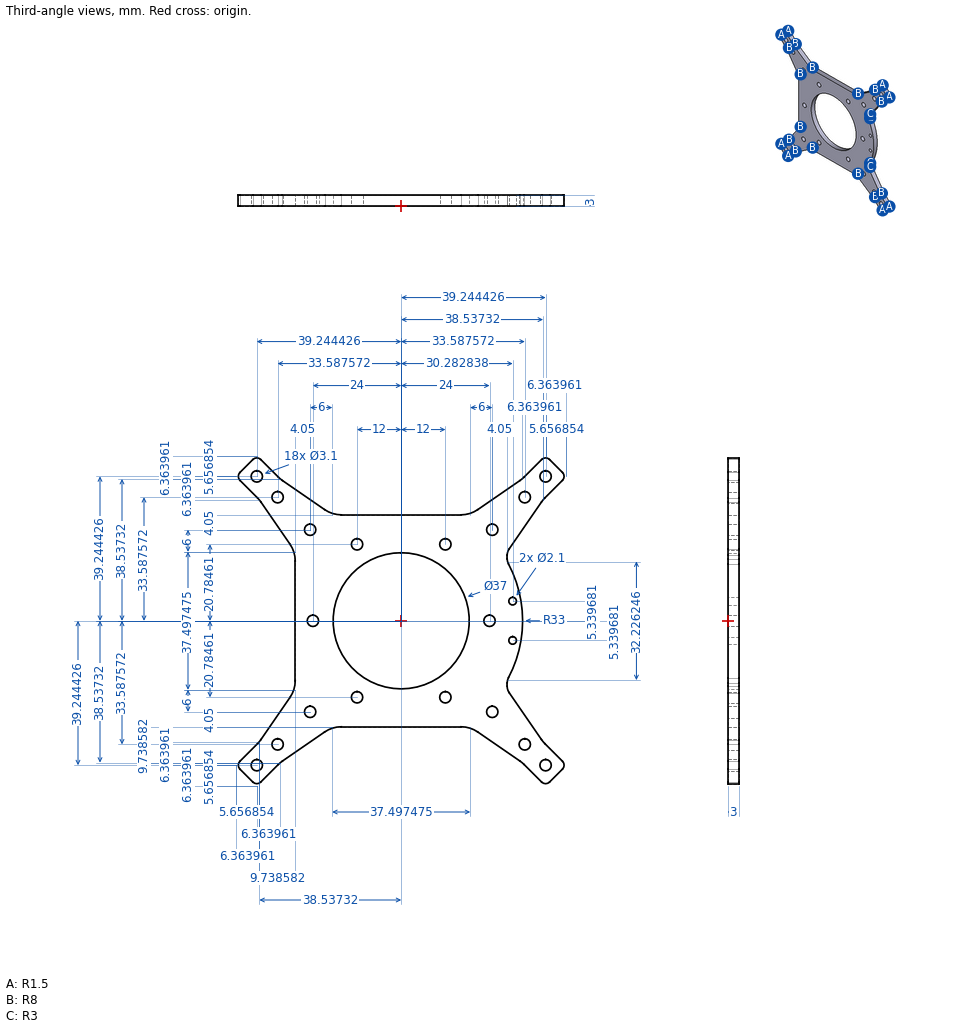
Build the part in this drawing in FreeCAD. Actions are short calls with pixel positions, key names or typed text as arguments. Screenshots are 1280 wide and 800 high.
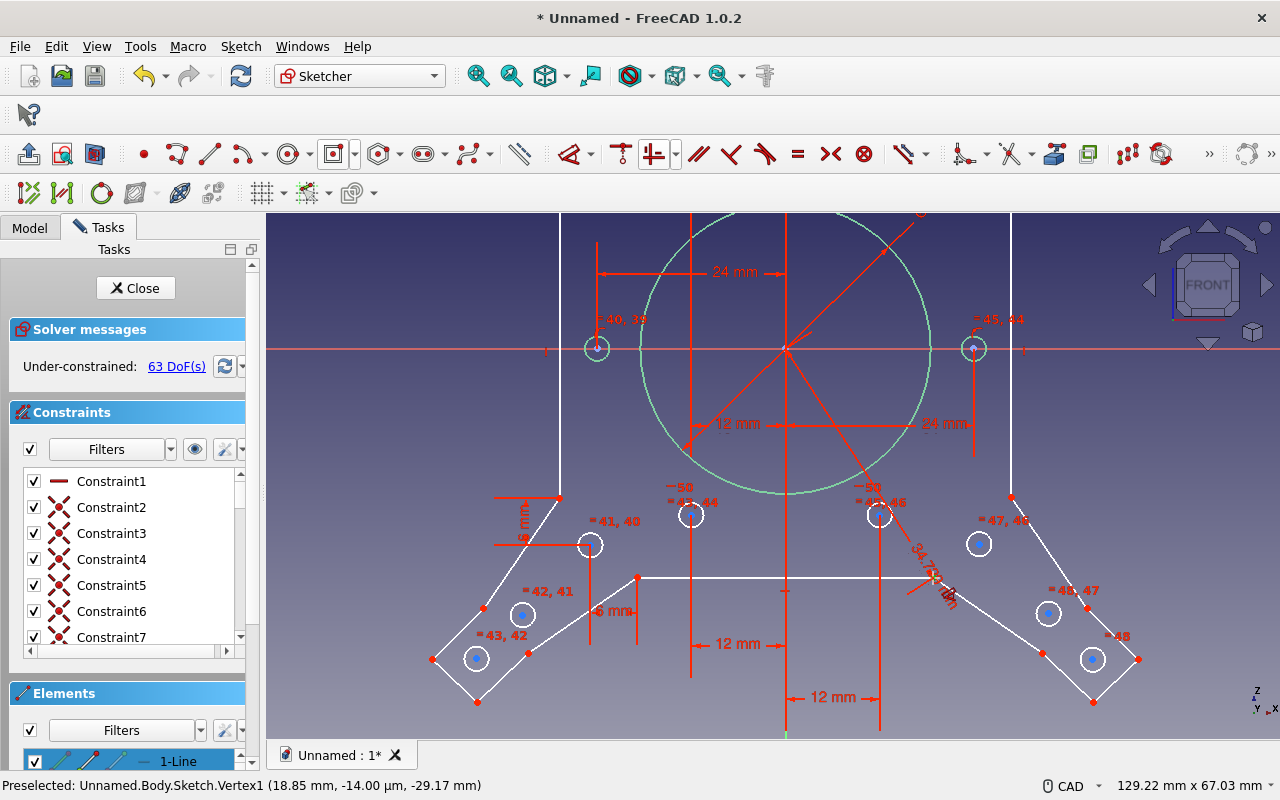
click(979, 544)
click(956, 612)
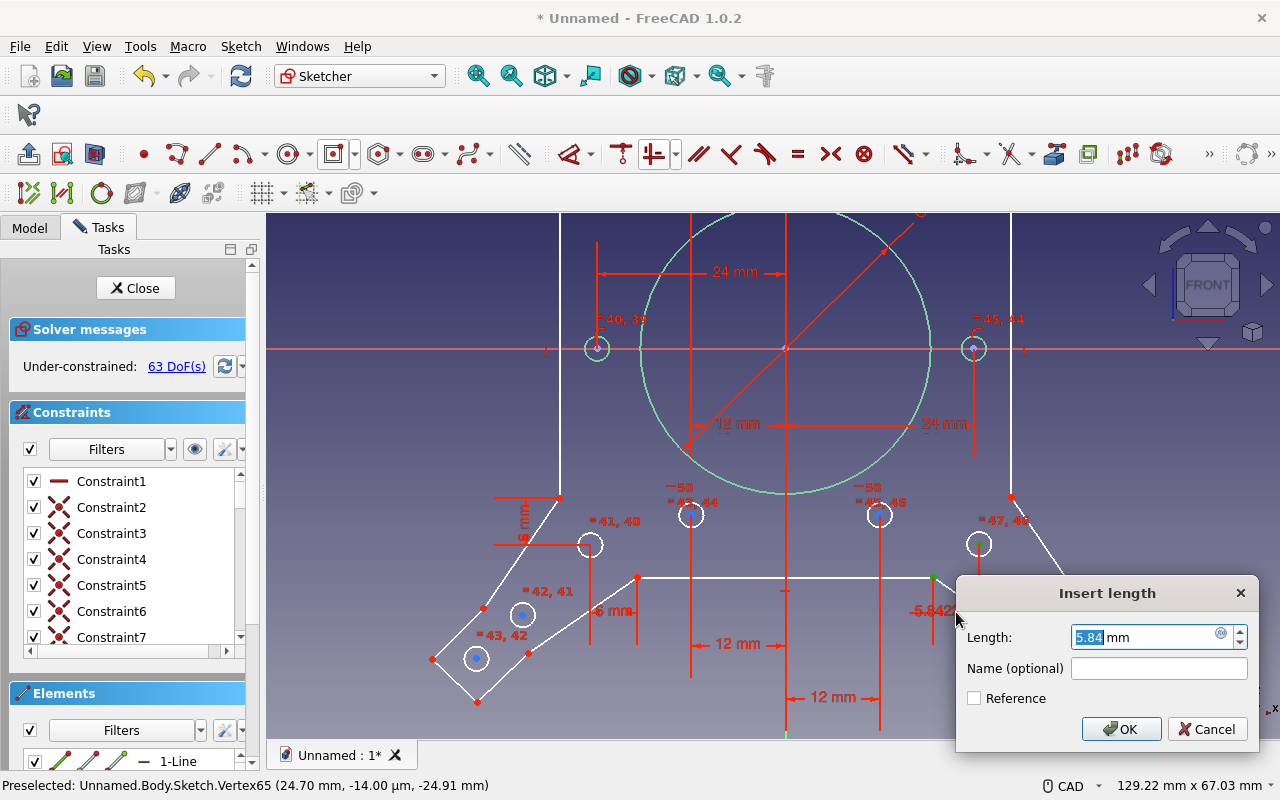
text(6)
key(Return)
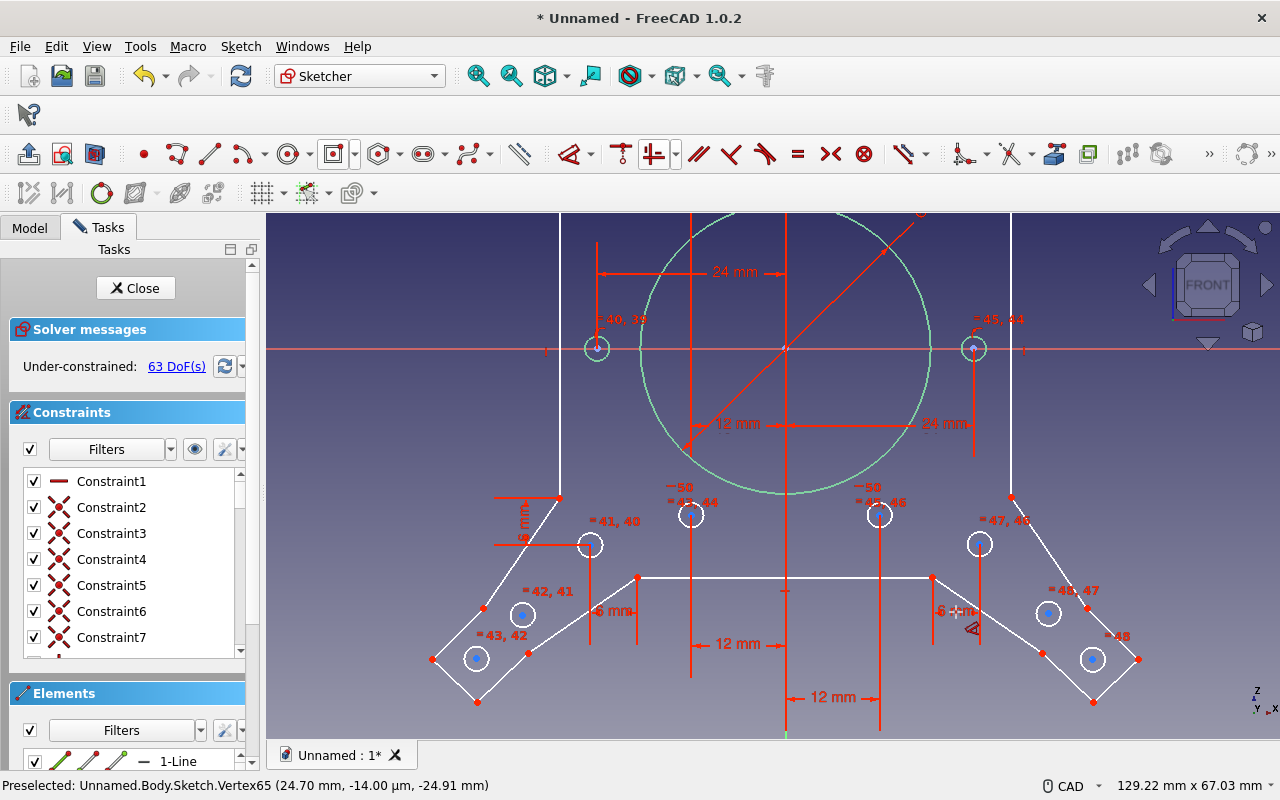
click(1011, 498)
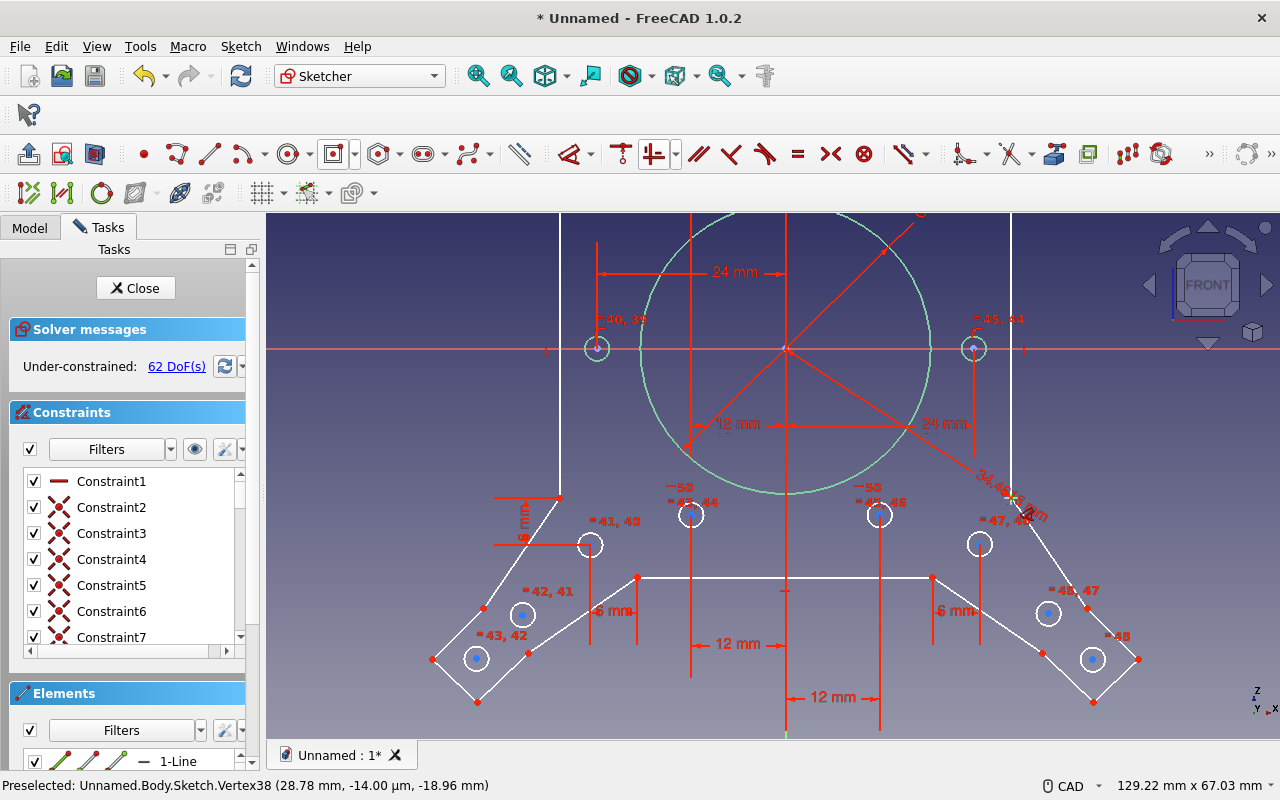
click(980, 544)
click(1045, 521)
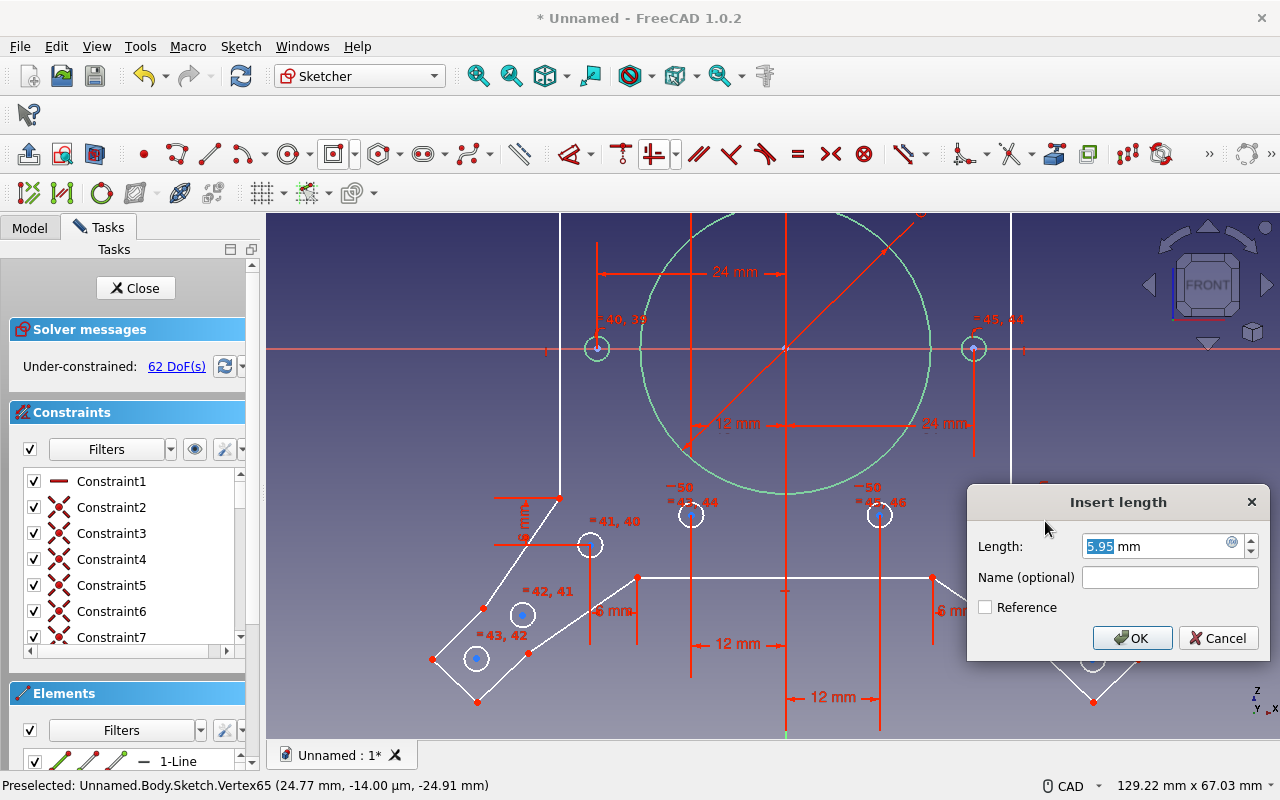
text(6)
key(Return)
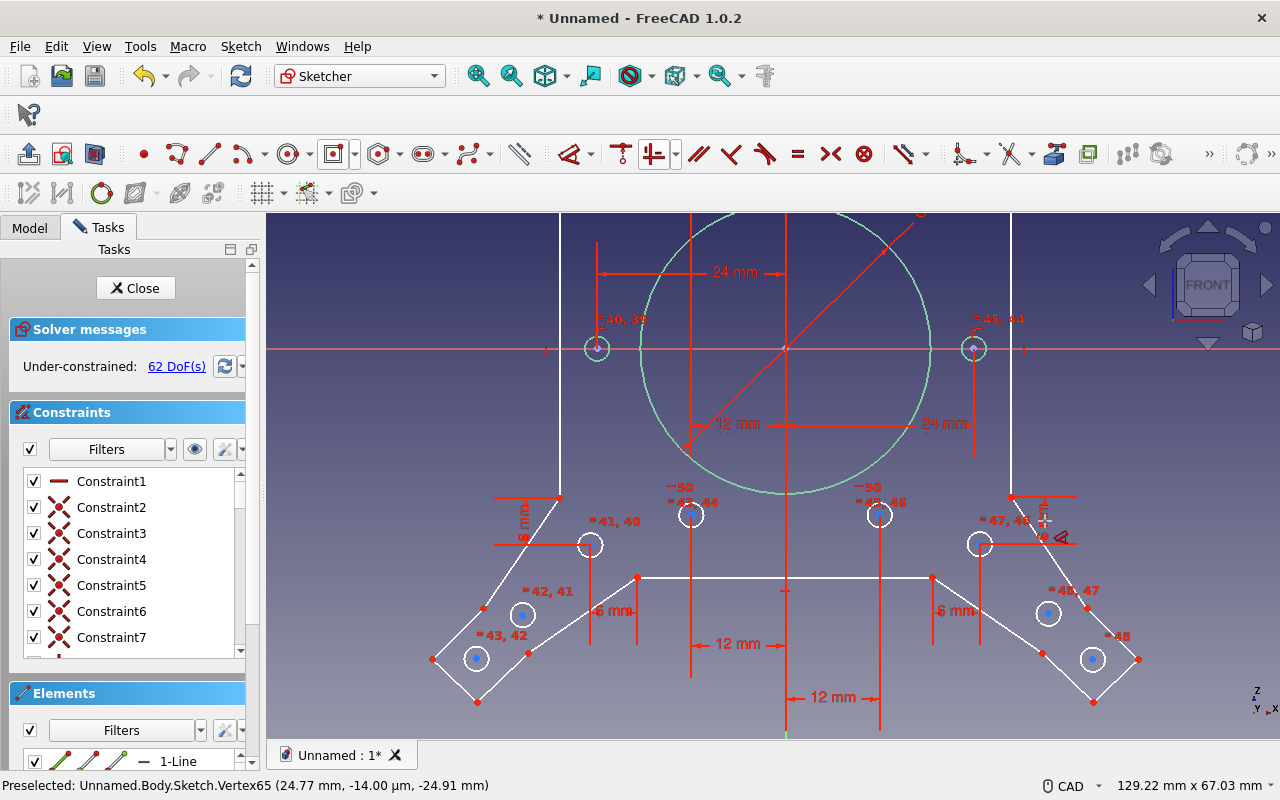
scroll(638, 580, down, 4)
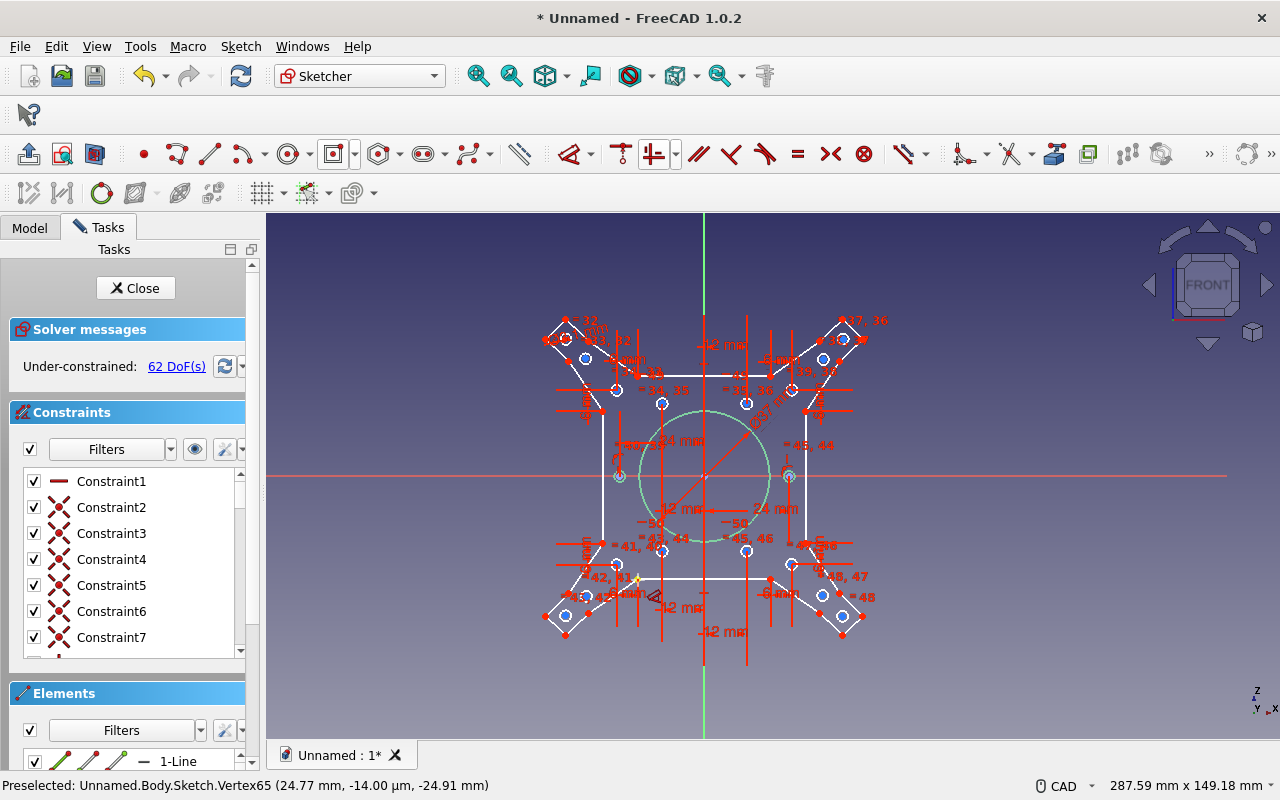
scroll(603, 411, up, 6)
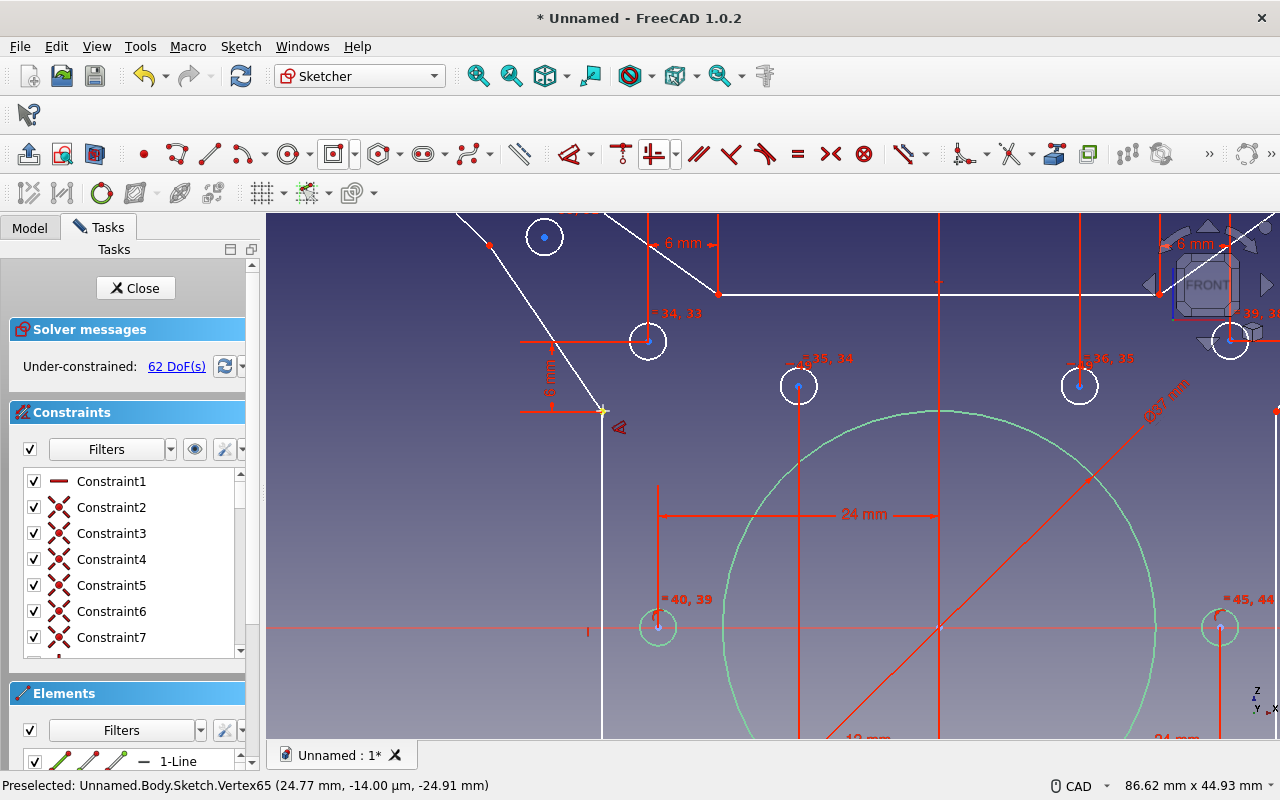
click(602, 412)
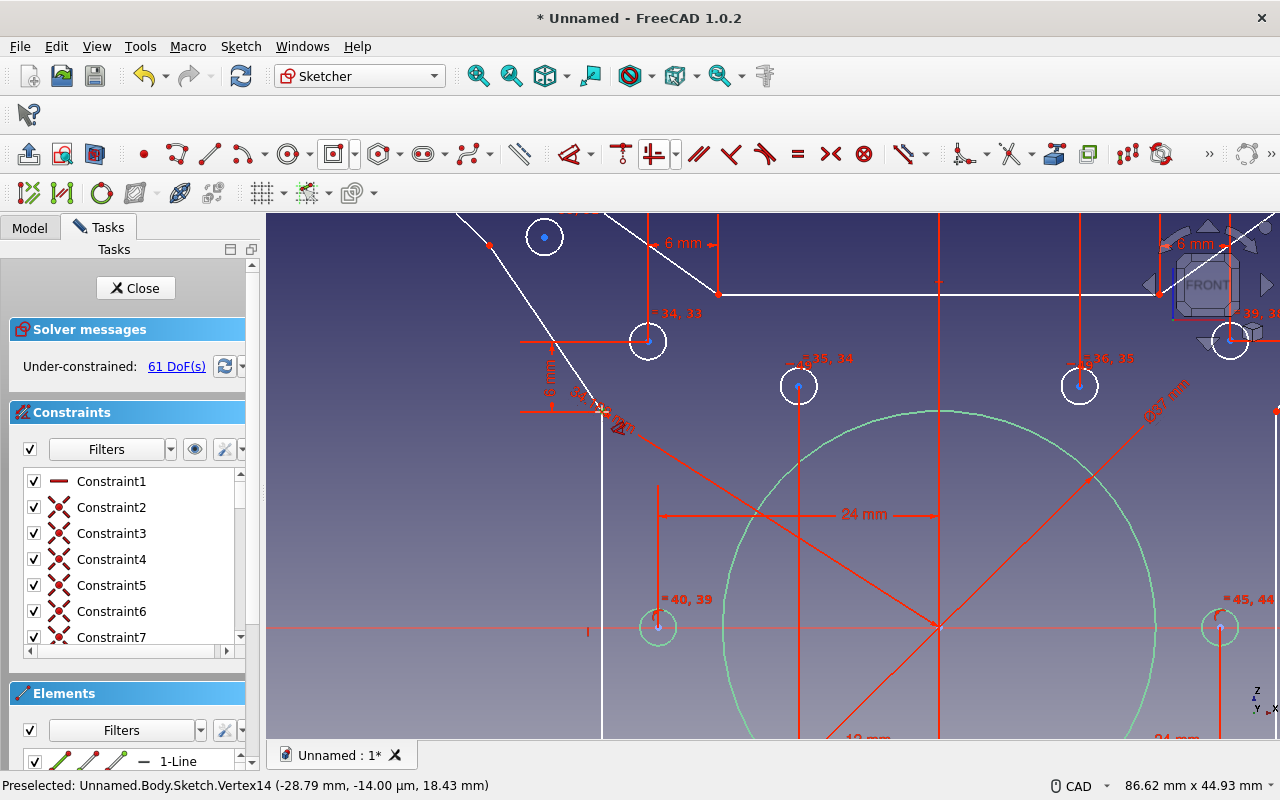
click(648, 342)
click(625, 308)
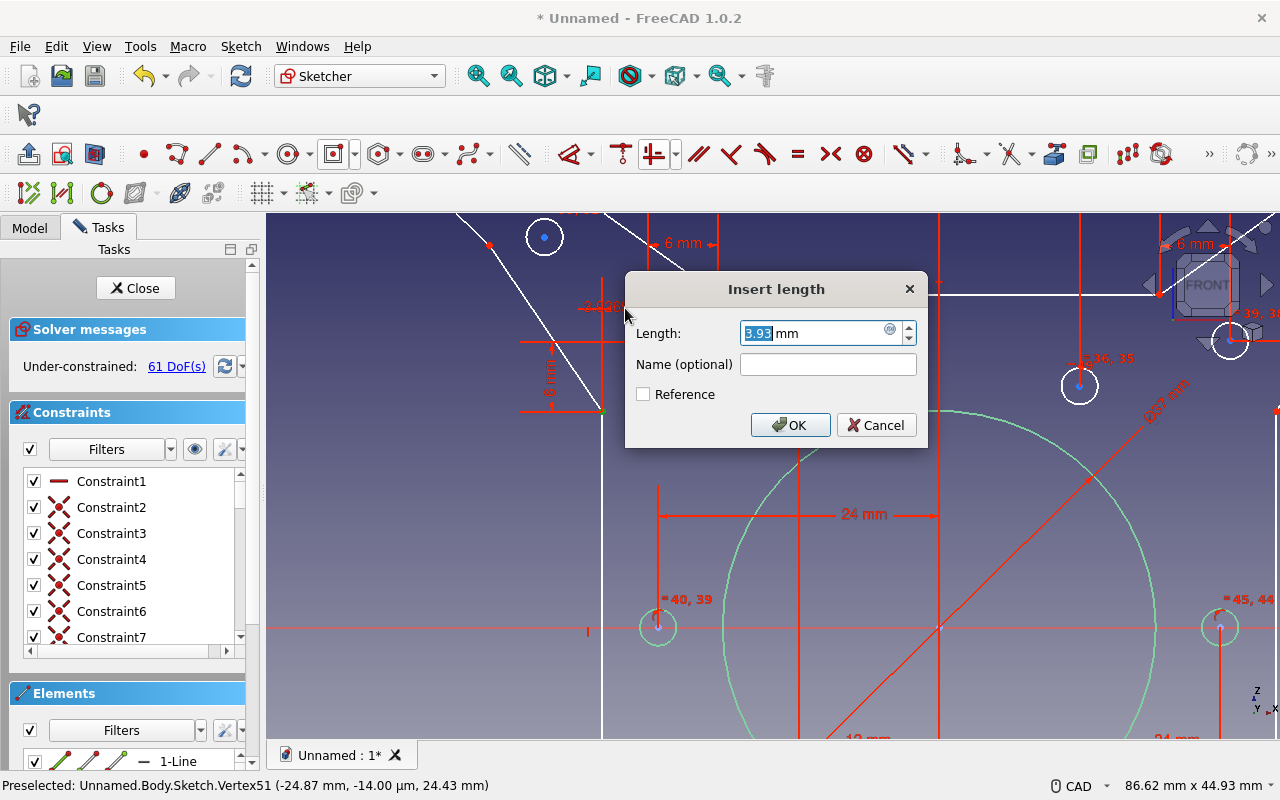
text(4.05)
key(Return)